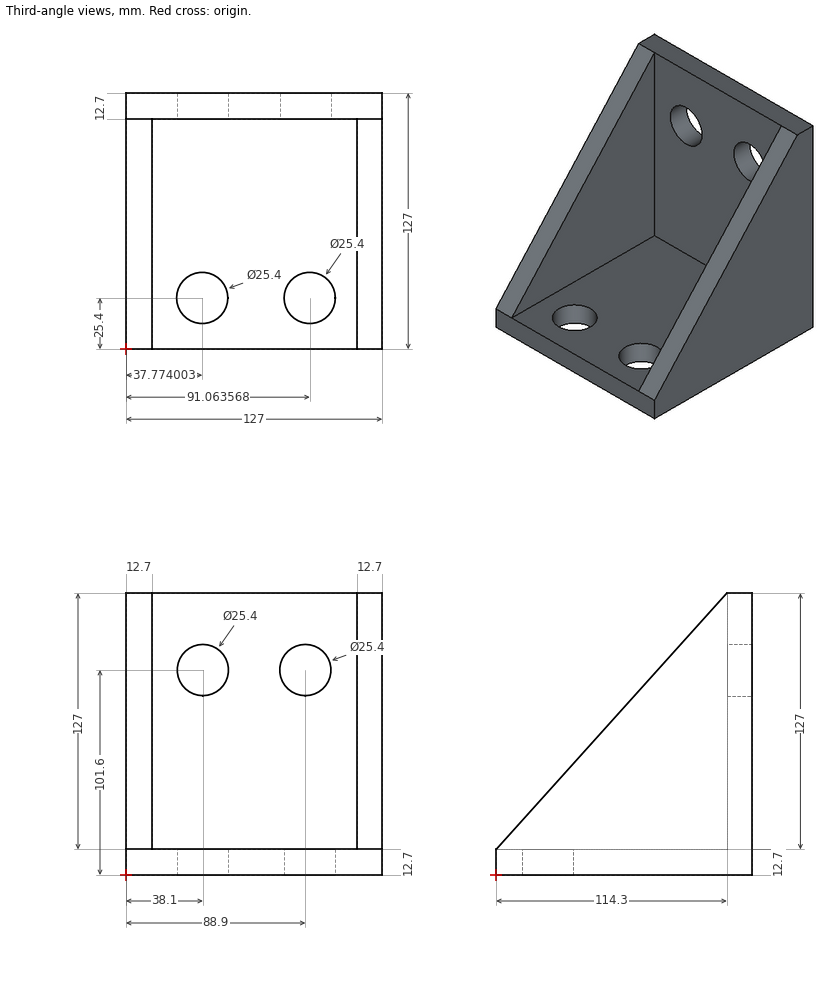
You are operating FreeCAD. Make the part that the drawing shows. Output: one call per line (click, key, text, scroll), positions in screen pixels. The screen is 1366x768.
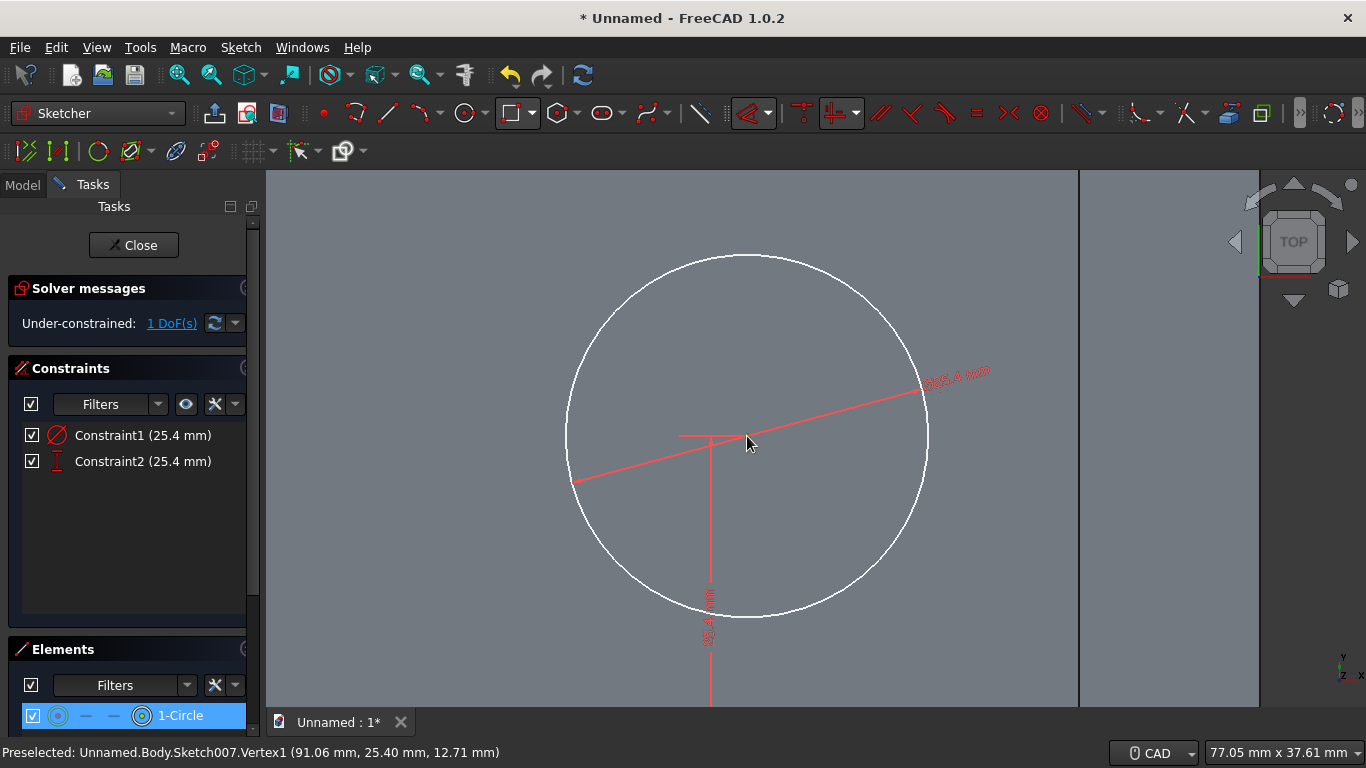
key(l)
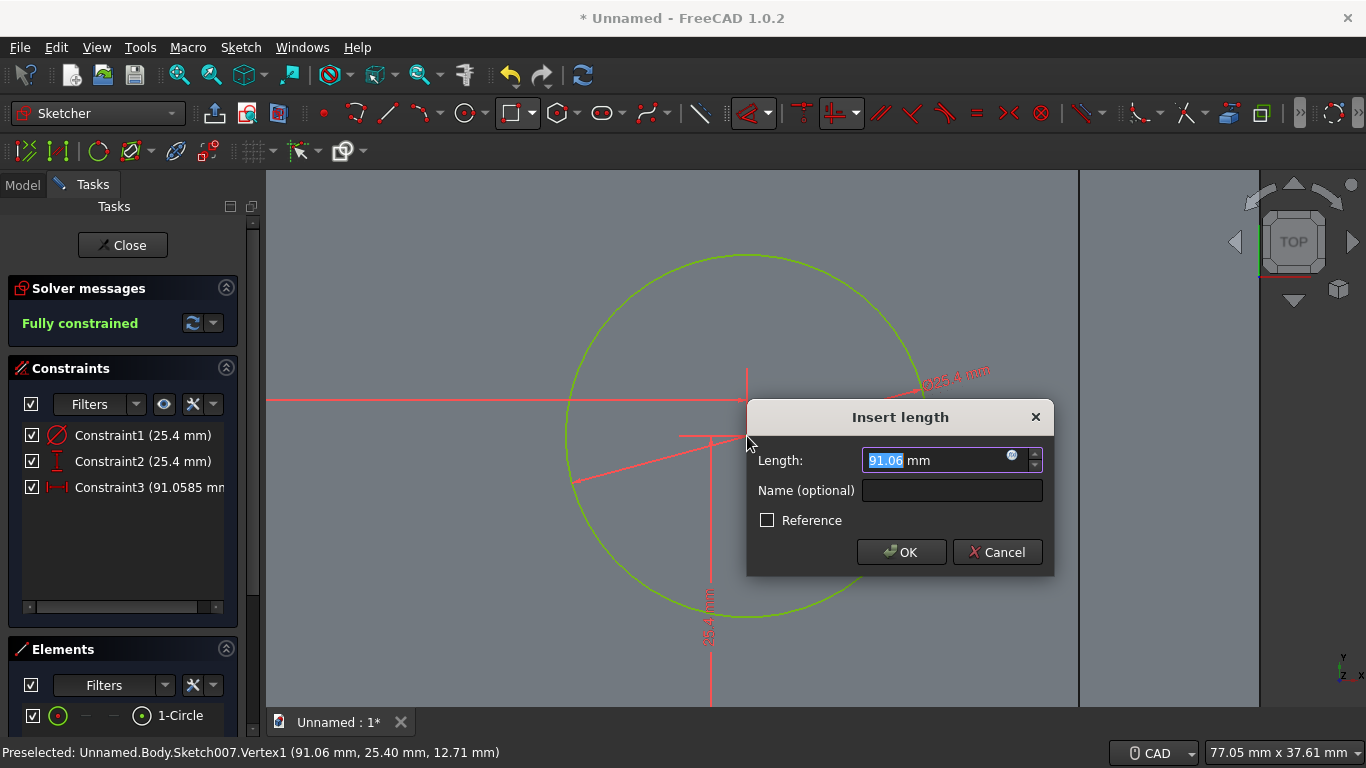
text(91.063568)
key(Return)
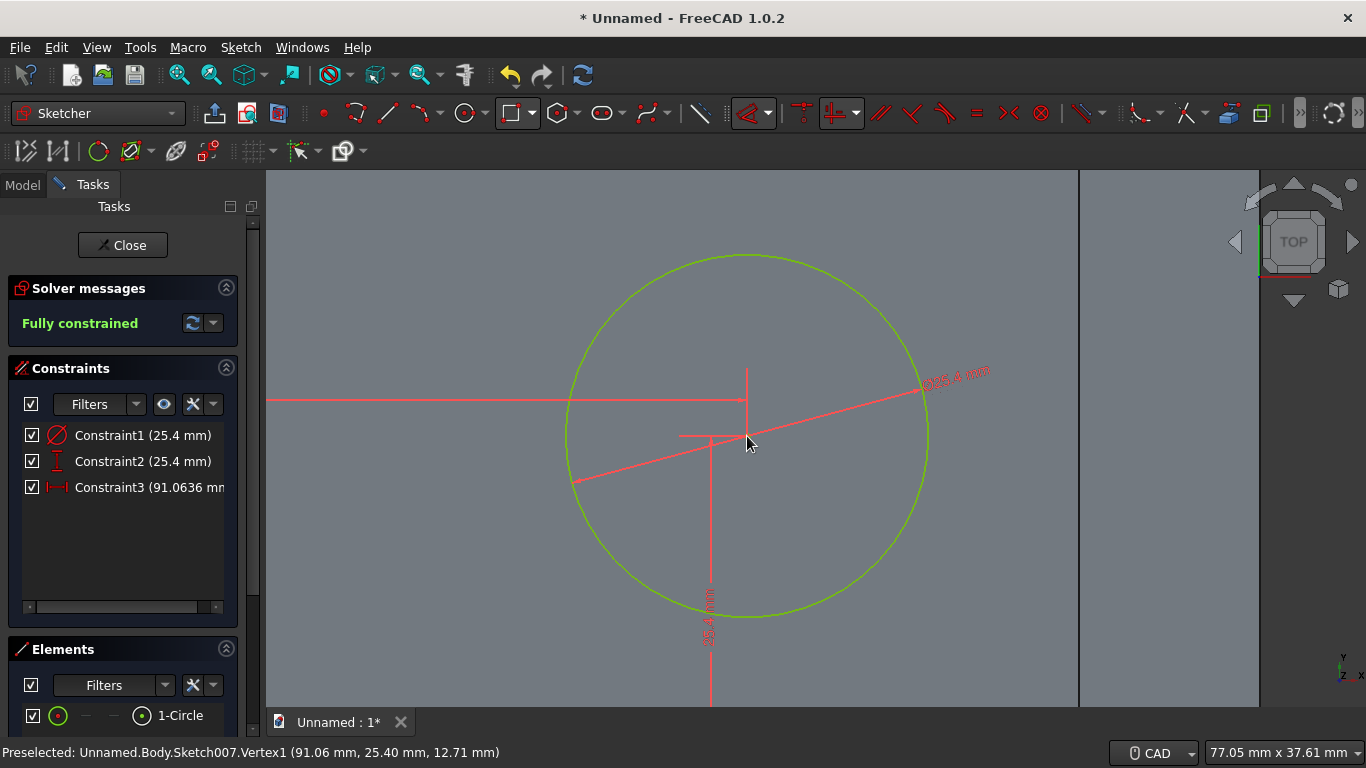
click(123, 245)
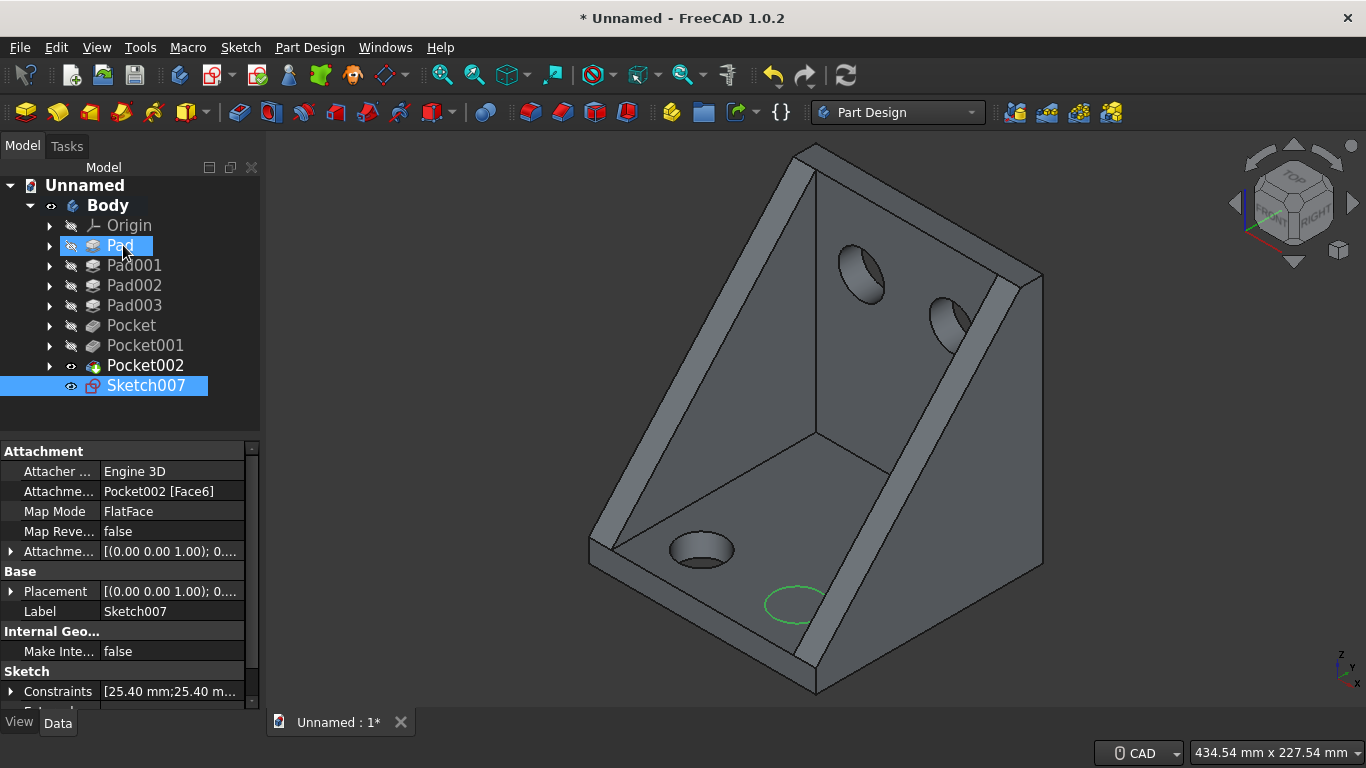
click(240, 112)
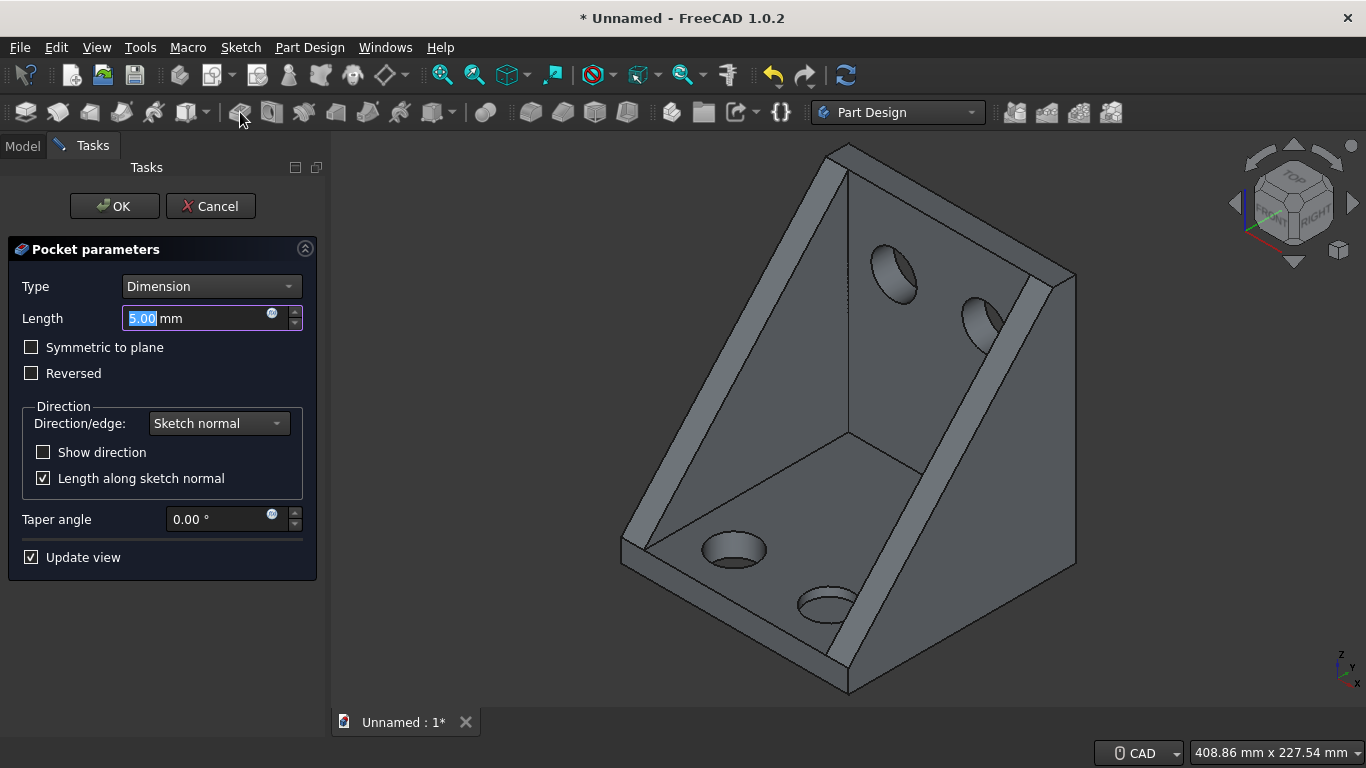
text(12.7)
key(Tab)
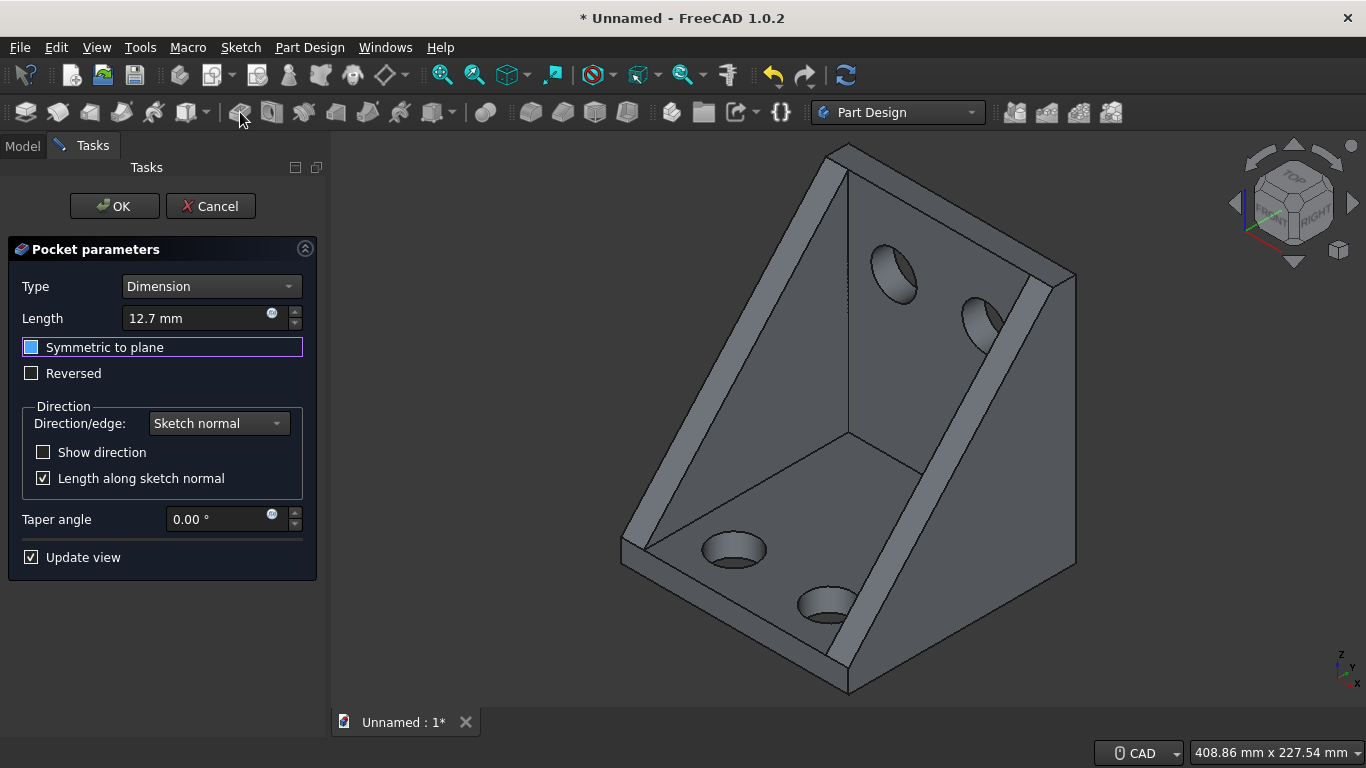
click(115, 206)